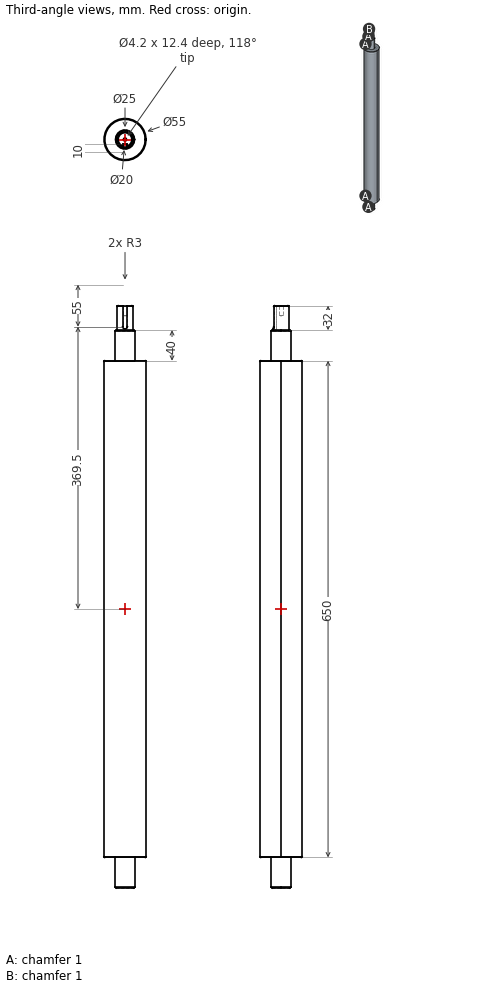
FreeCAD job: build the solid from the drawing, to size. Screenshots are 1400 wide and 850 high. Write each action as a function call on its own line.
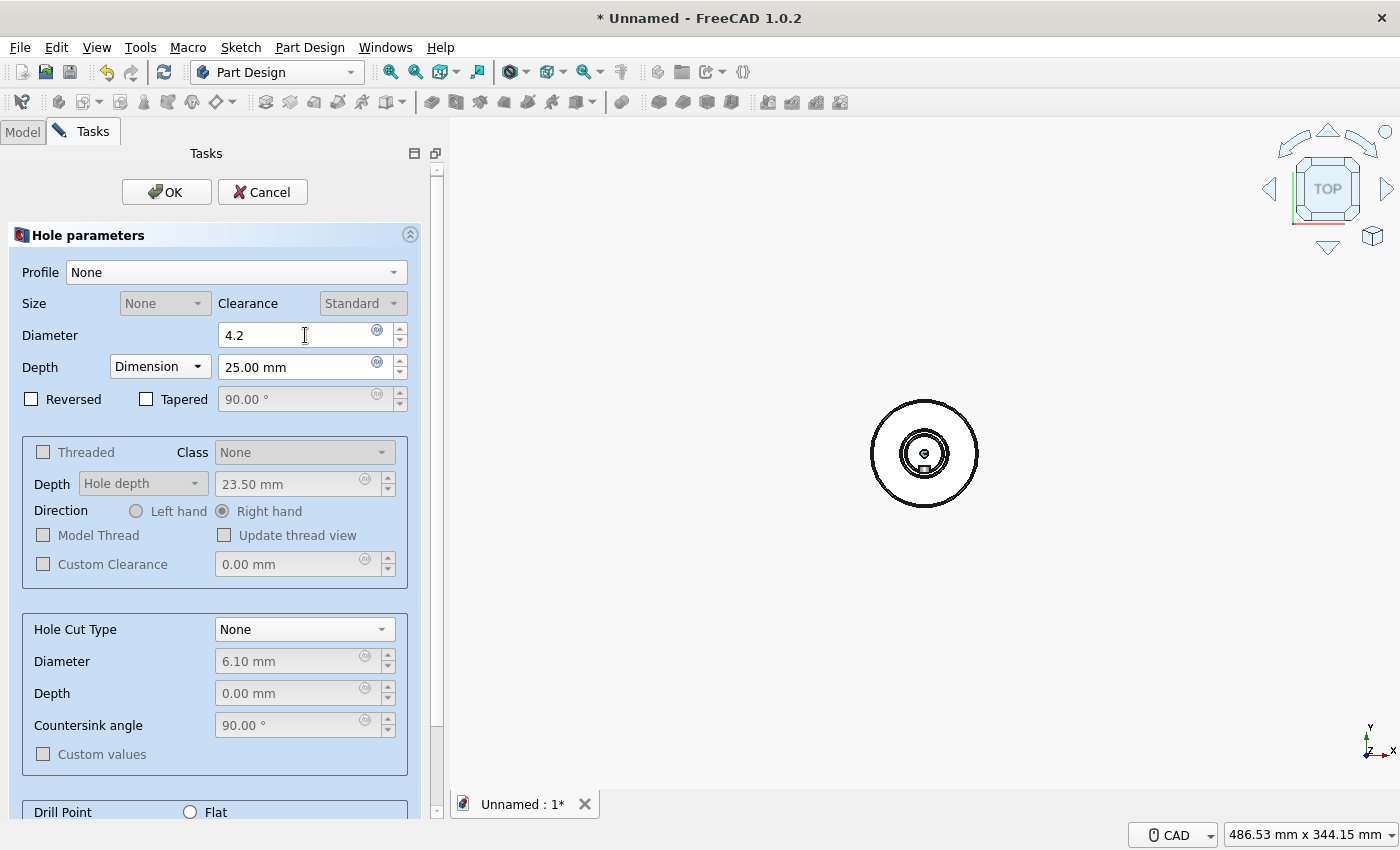
triple_click(305, 367)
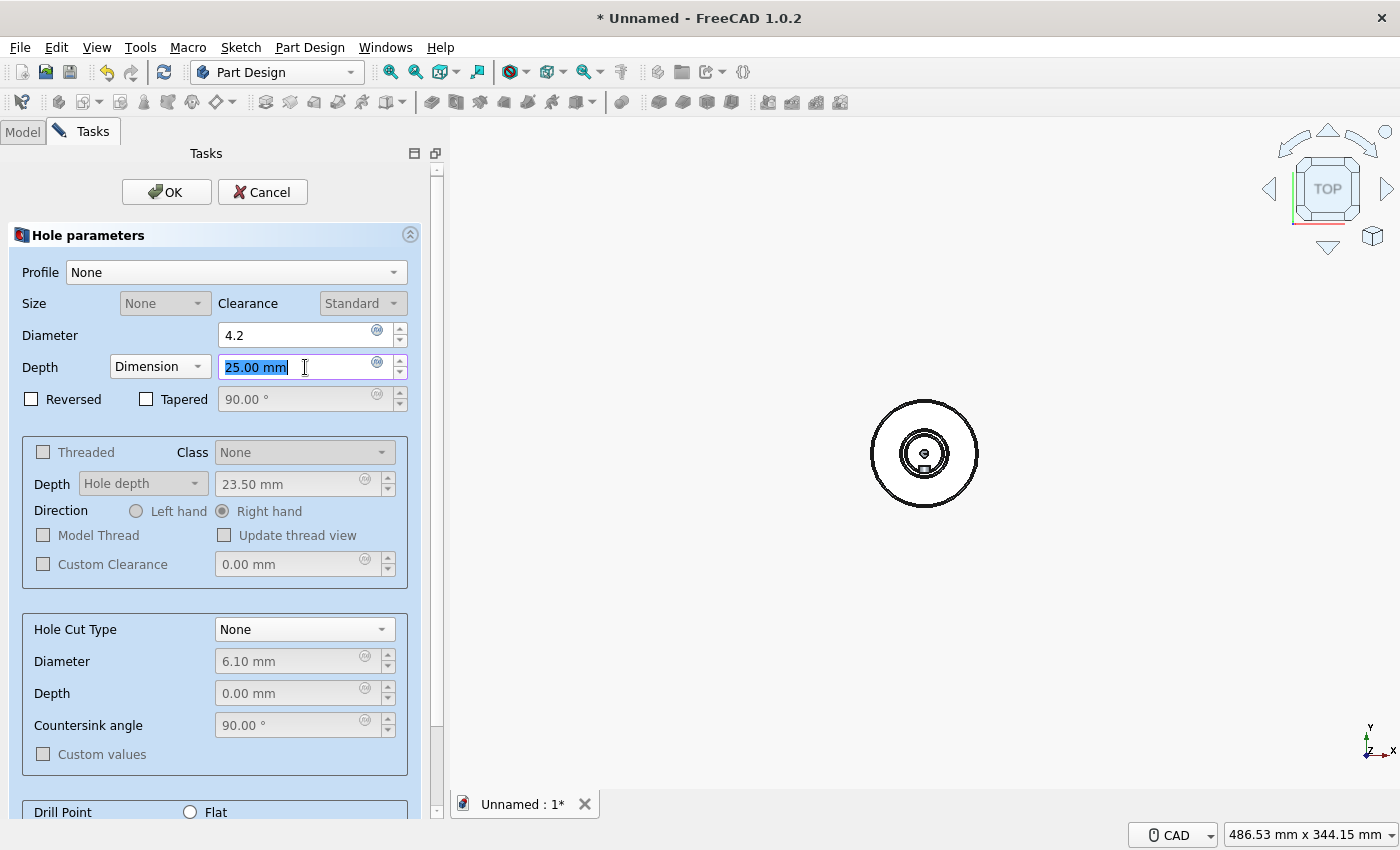
text(12.4)
key(Tab)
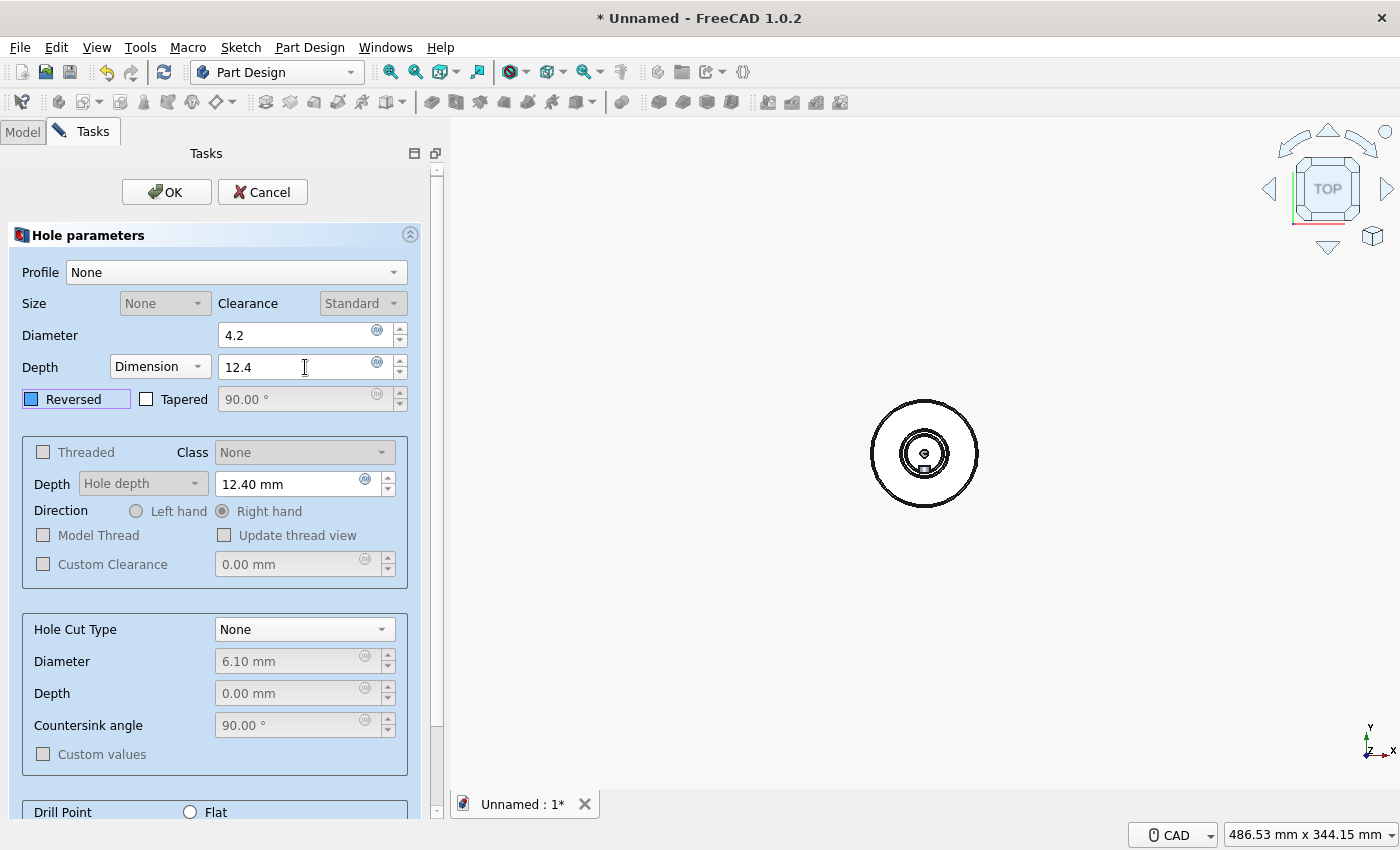
click(167, 192)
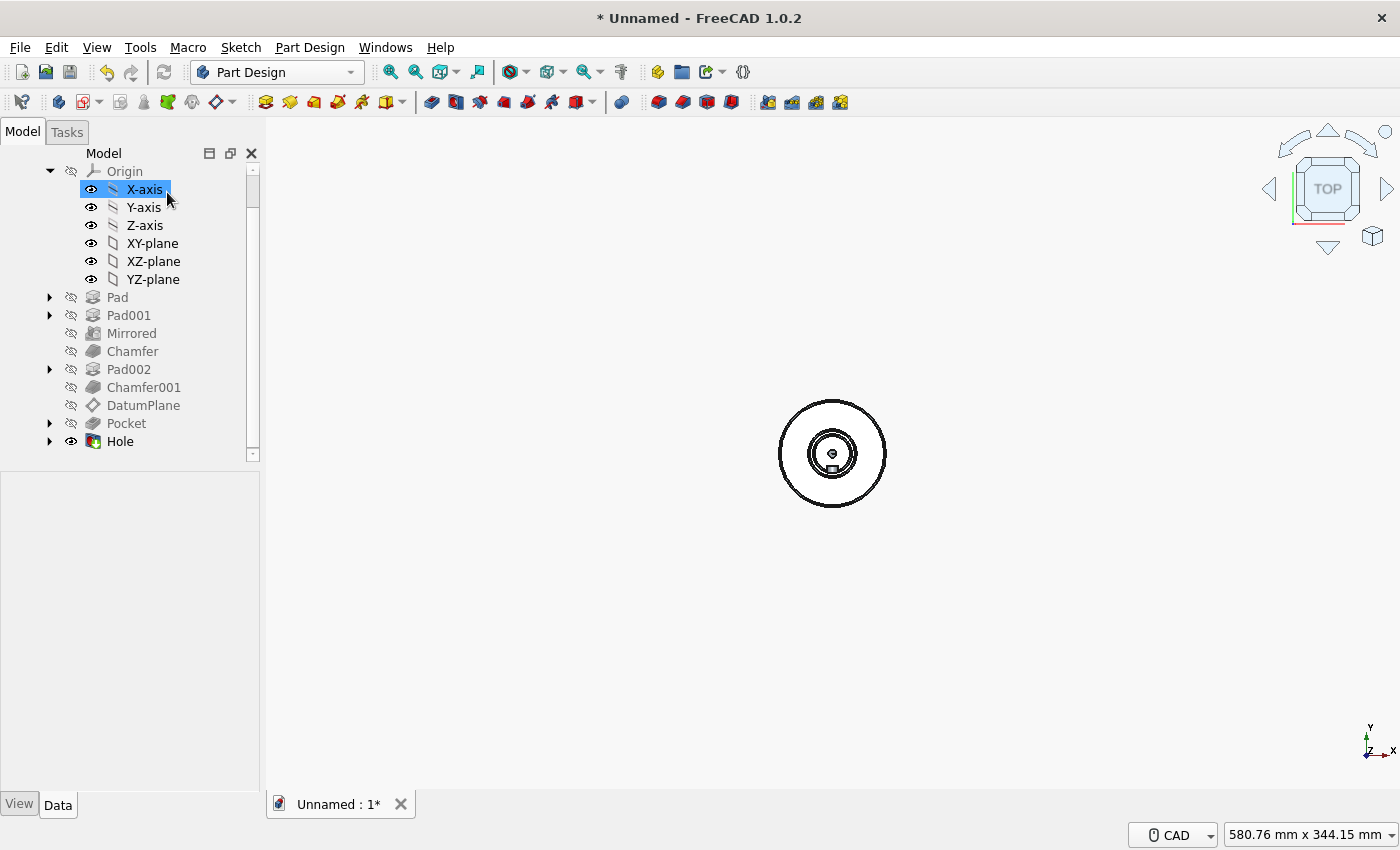
key(0)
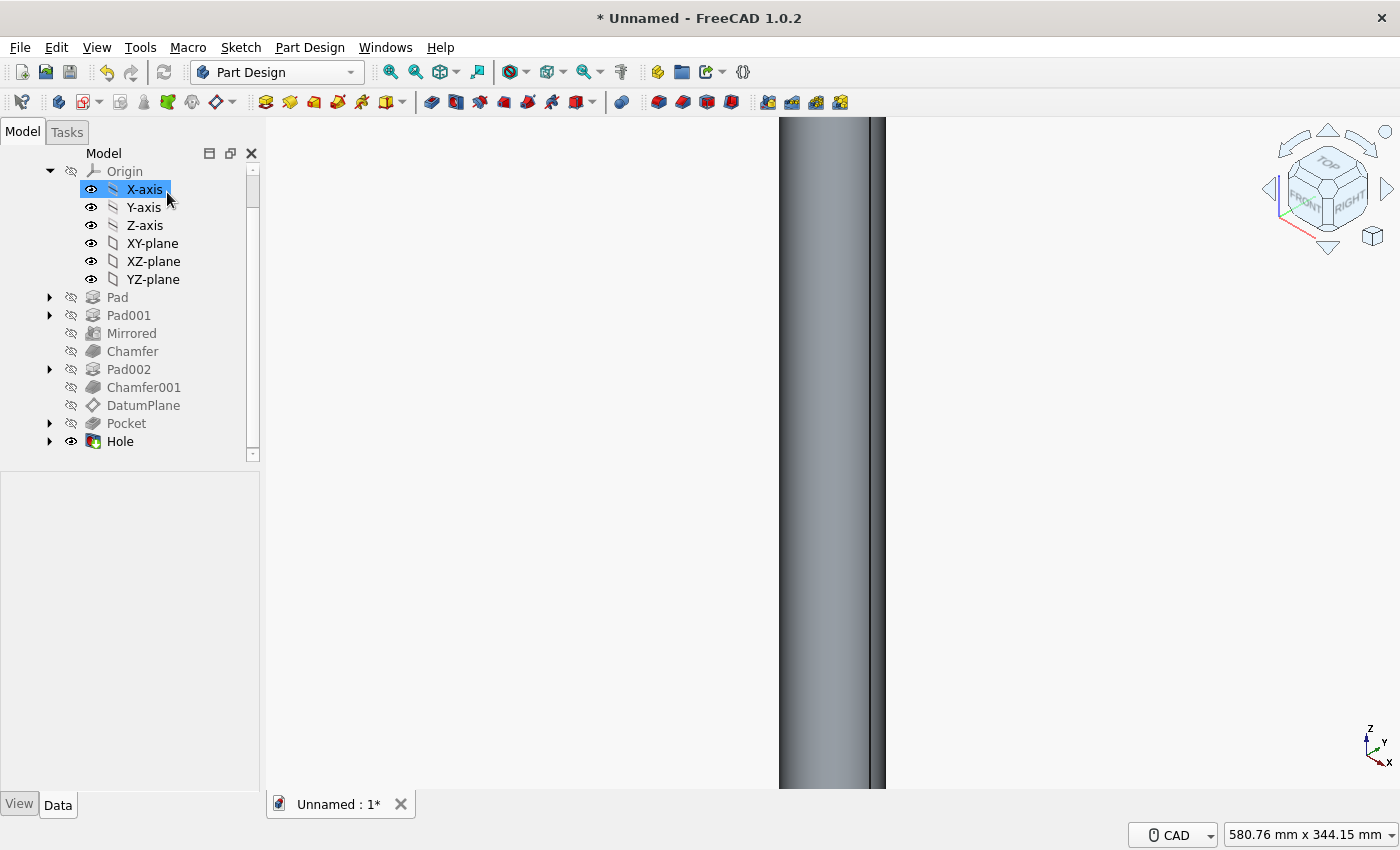
click(392, 72)